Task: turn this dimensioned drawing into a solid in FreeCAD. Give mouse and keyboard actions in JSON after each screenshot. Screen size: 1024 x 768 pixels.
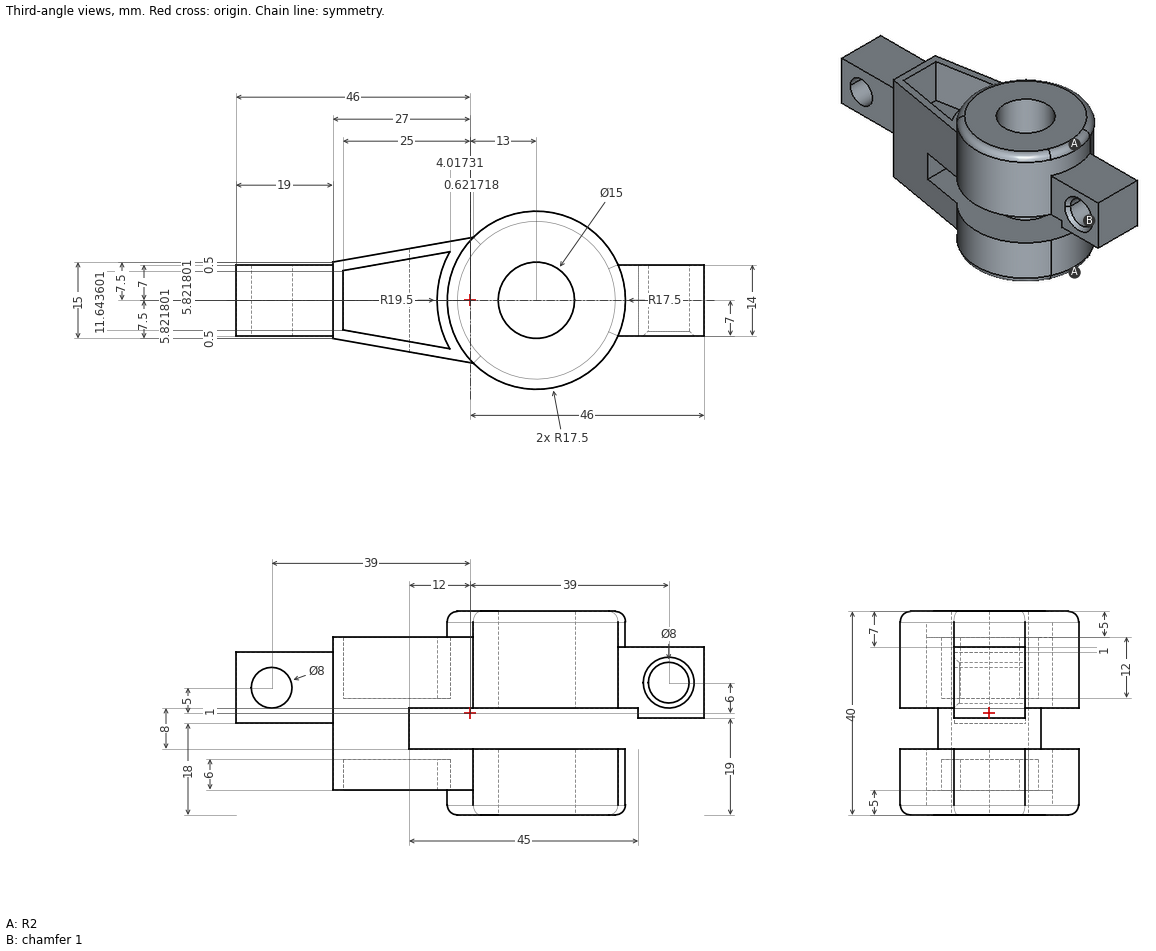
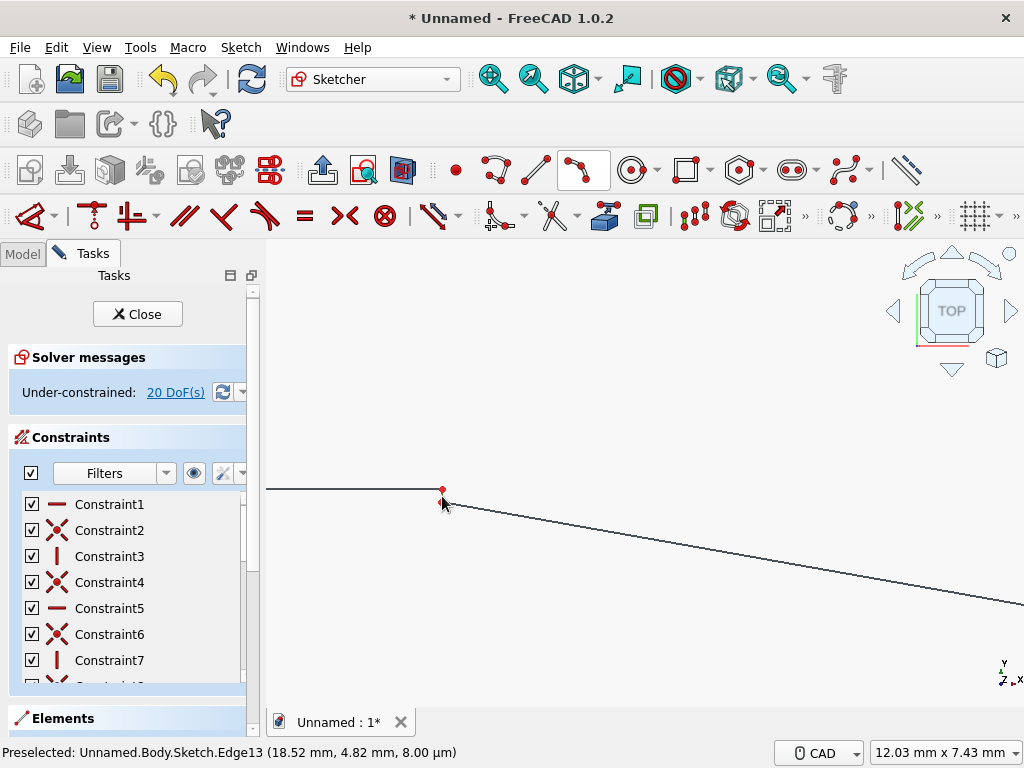
{"action": "left_click", "coordinate": [158, 216]}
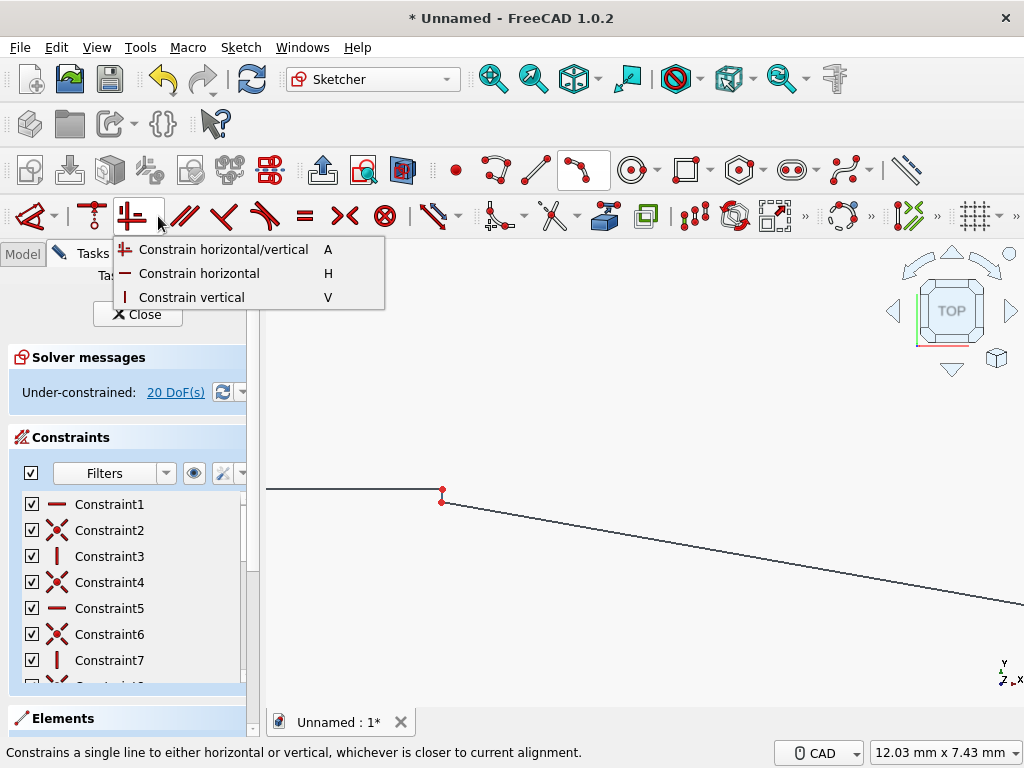
{"action": "left_click", "coordinate": [249, 297]}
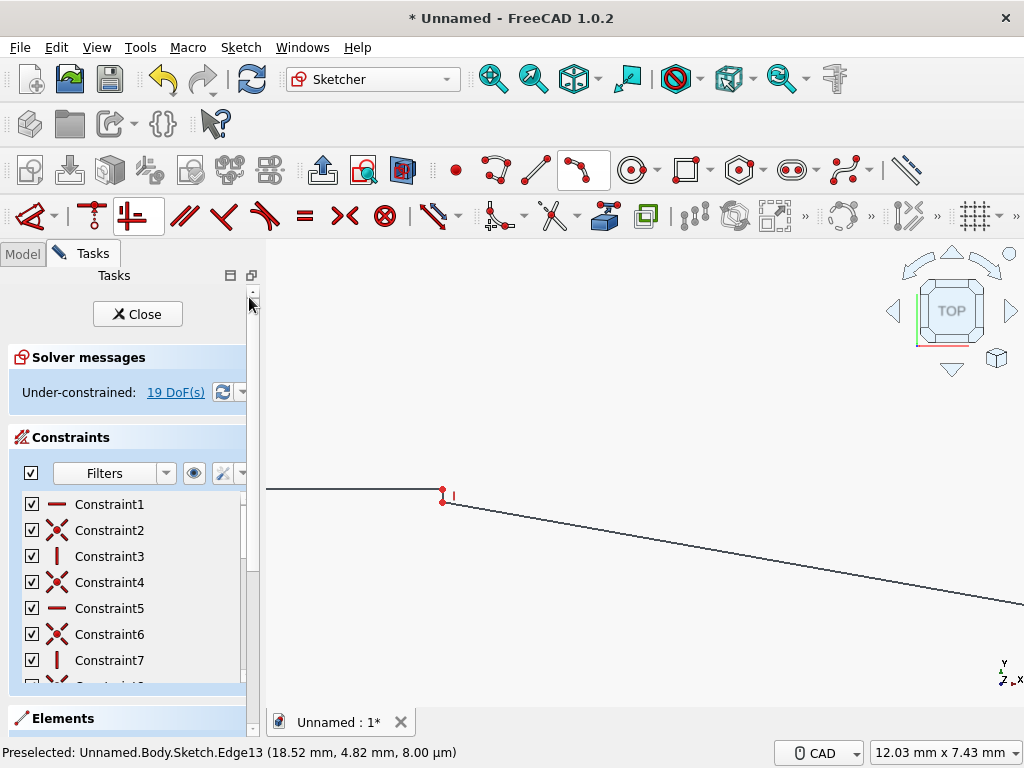
{"action": "scroll", "coordinate": [451, 509], "scroll_direction": "down", "scroll_amount": 13}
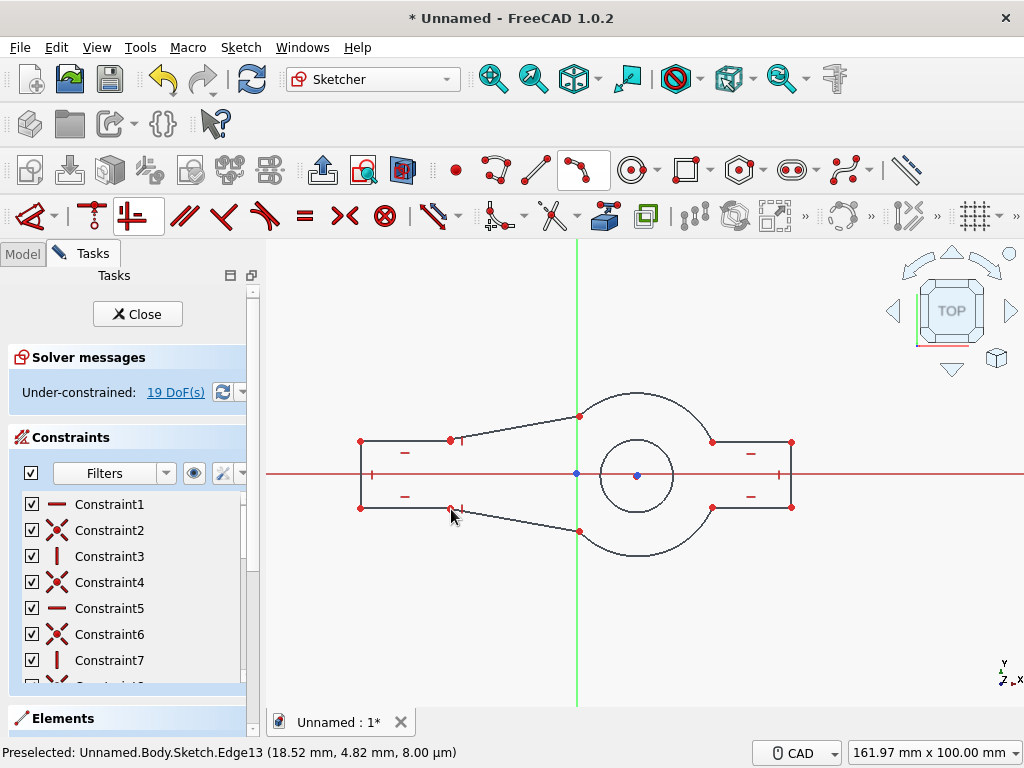
{"action": "left_click", "coordinate": [662, 450]}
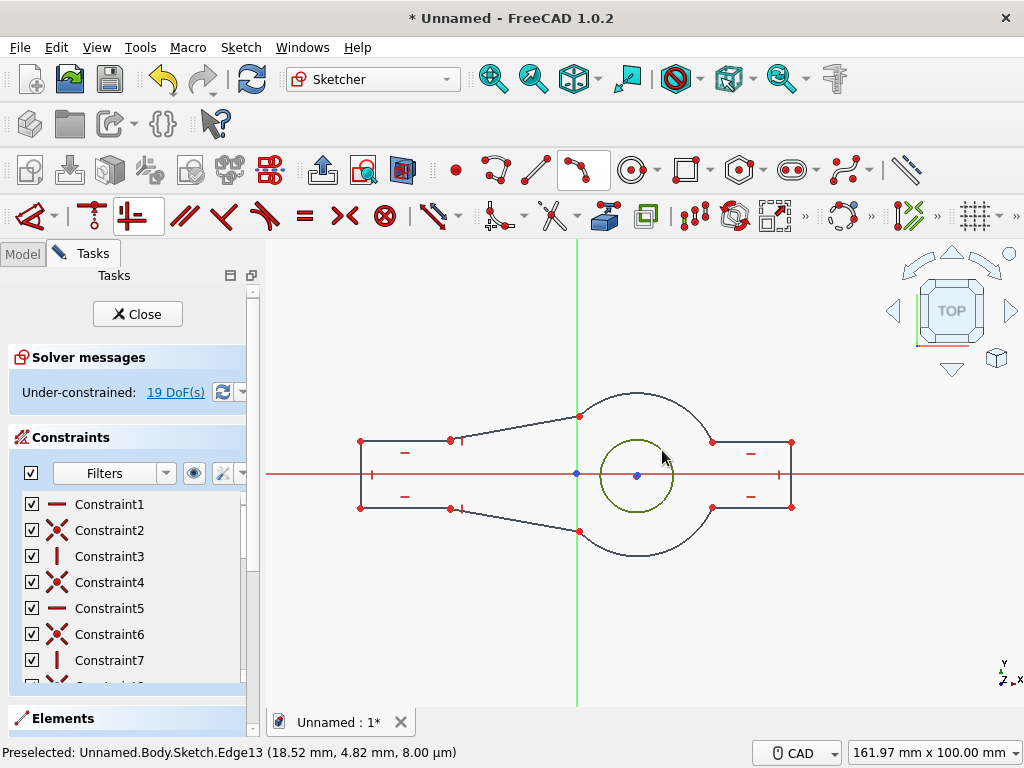
{"action": "left_click", "coordinate": [621, 555]}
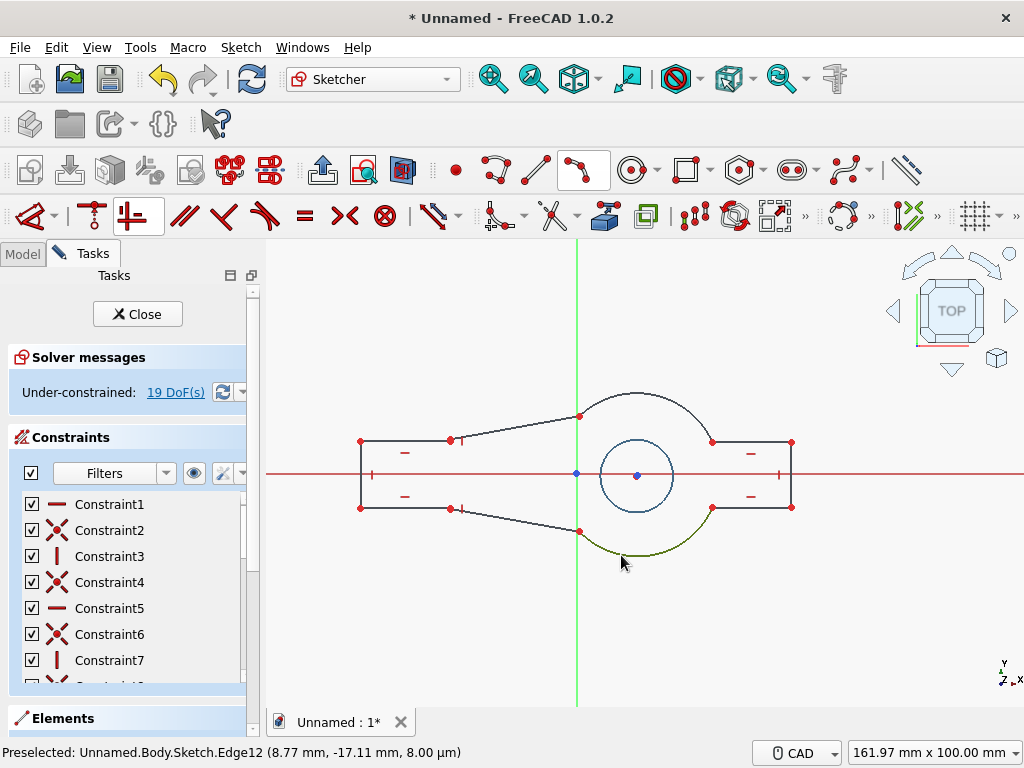
{"action": "left_click", "coordinate": [92, 216]}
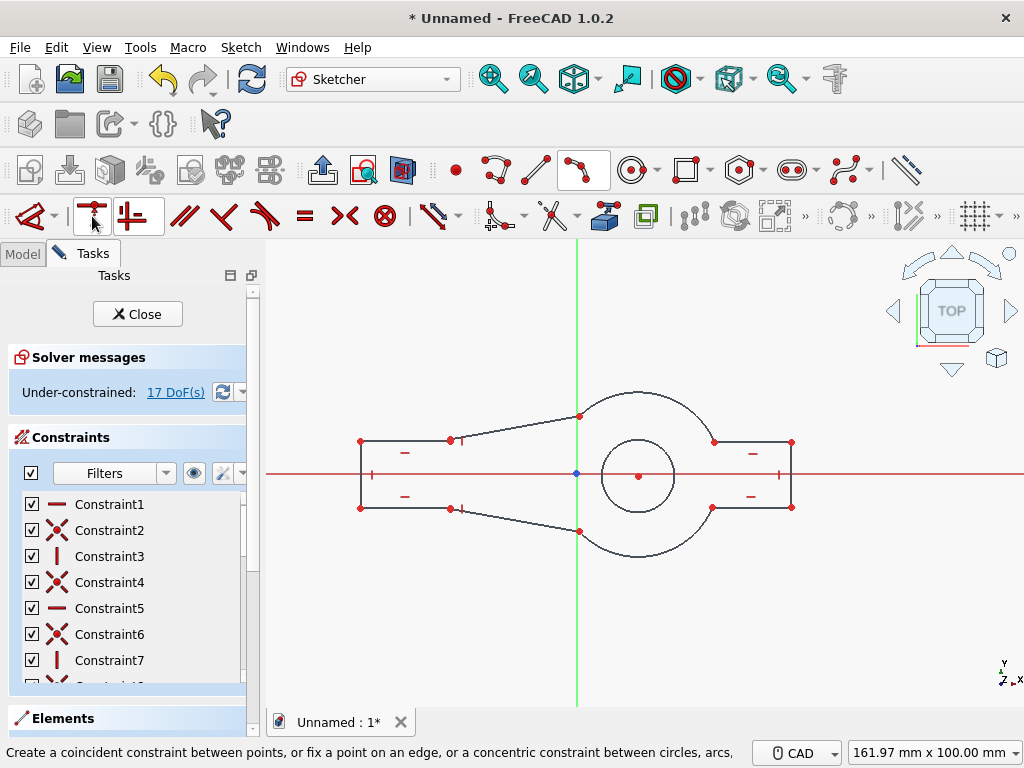
{"action": "left_click", "coordinate": [684, 406]}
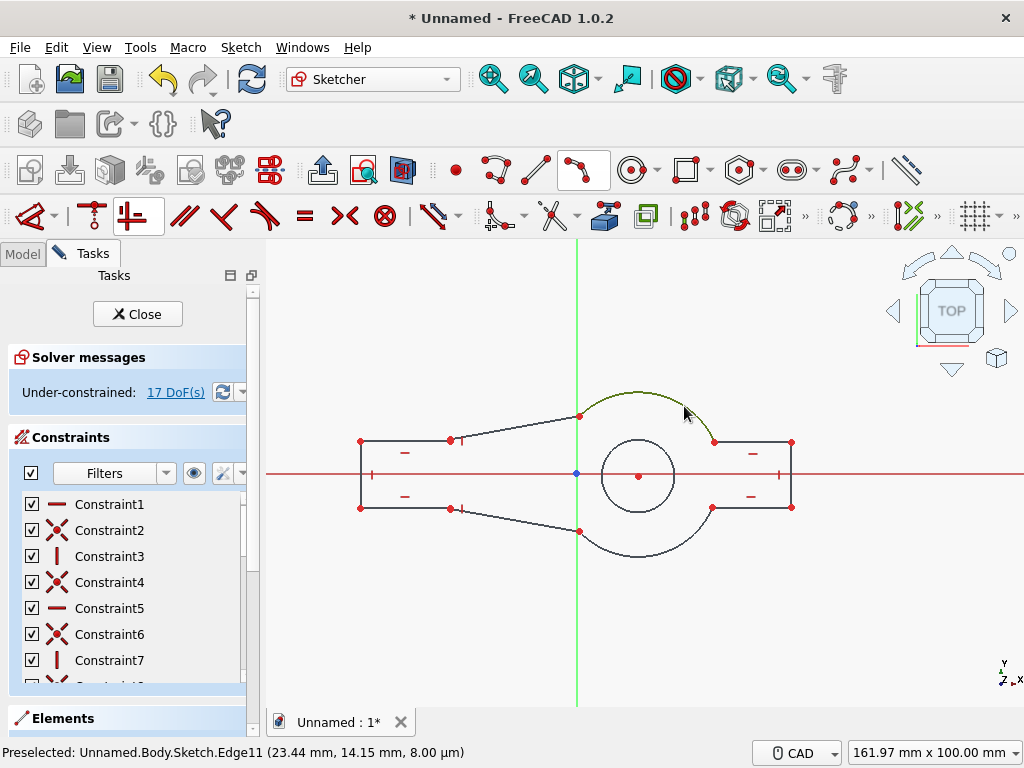
{"action": "left_click", "coordinate": [621, 555]}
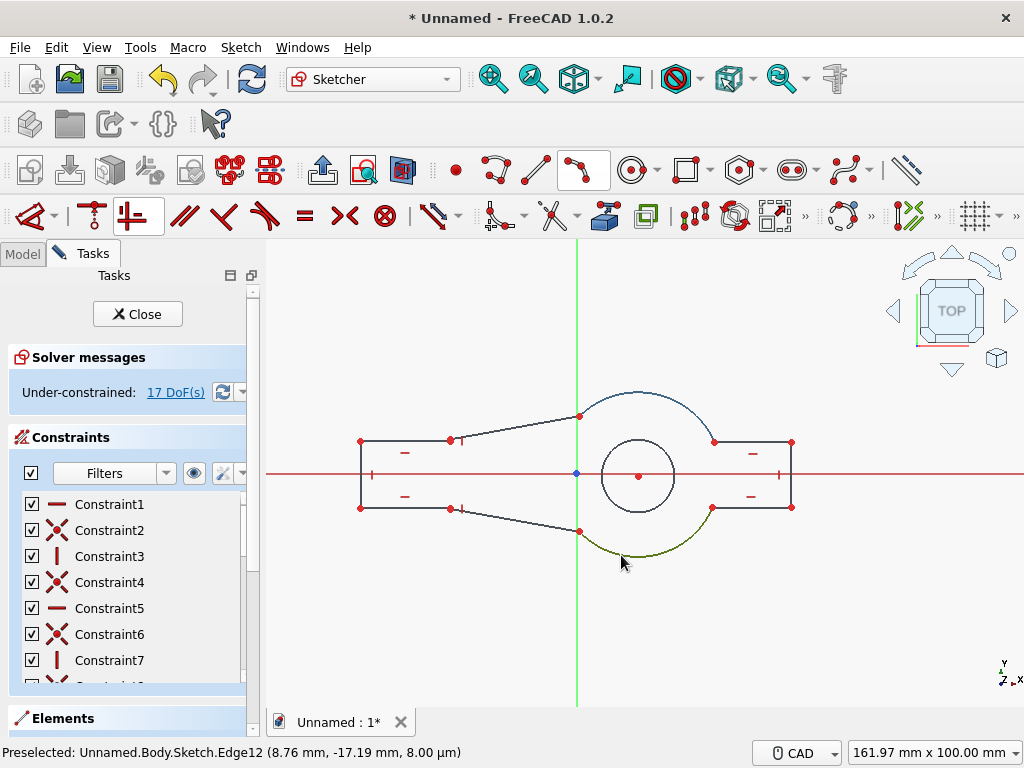
{"action": "left_click", "coordinate": [306, 216]}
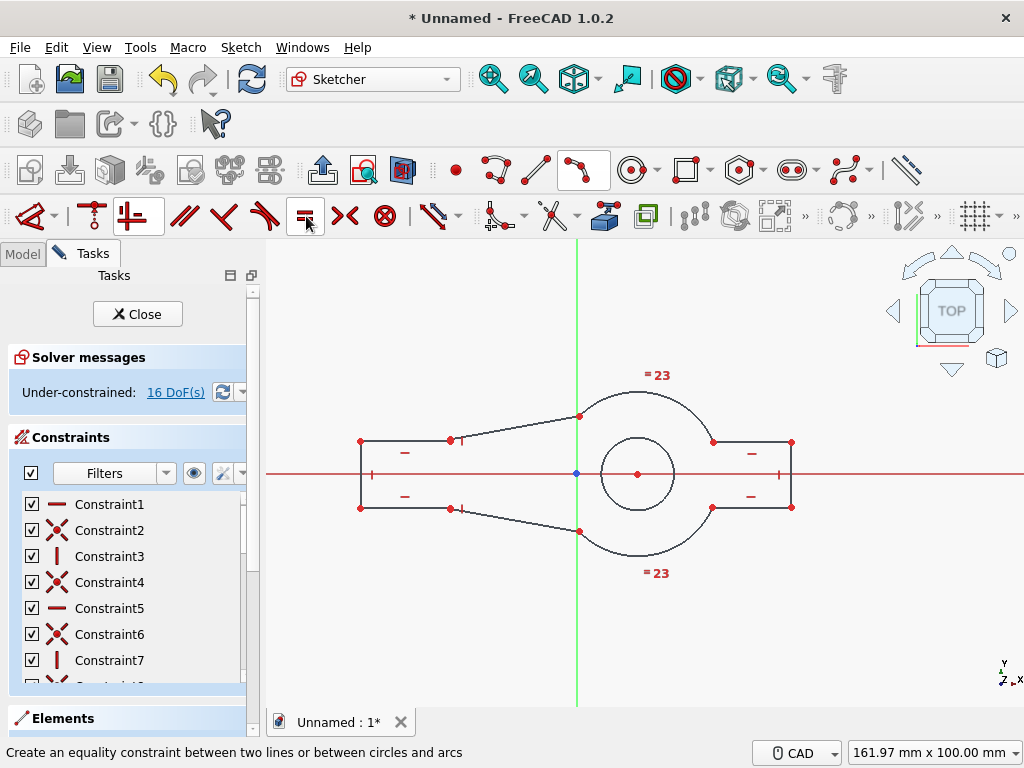
{"action": "left_click", "coordinate": [638, 474]}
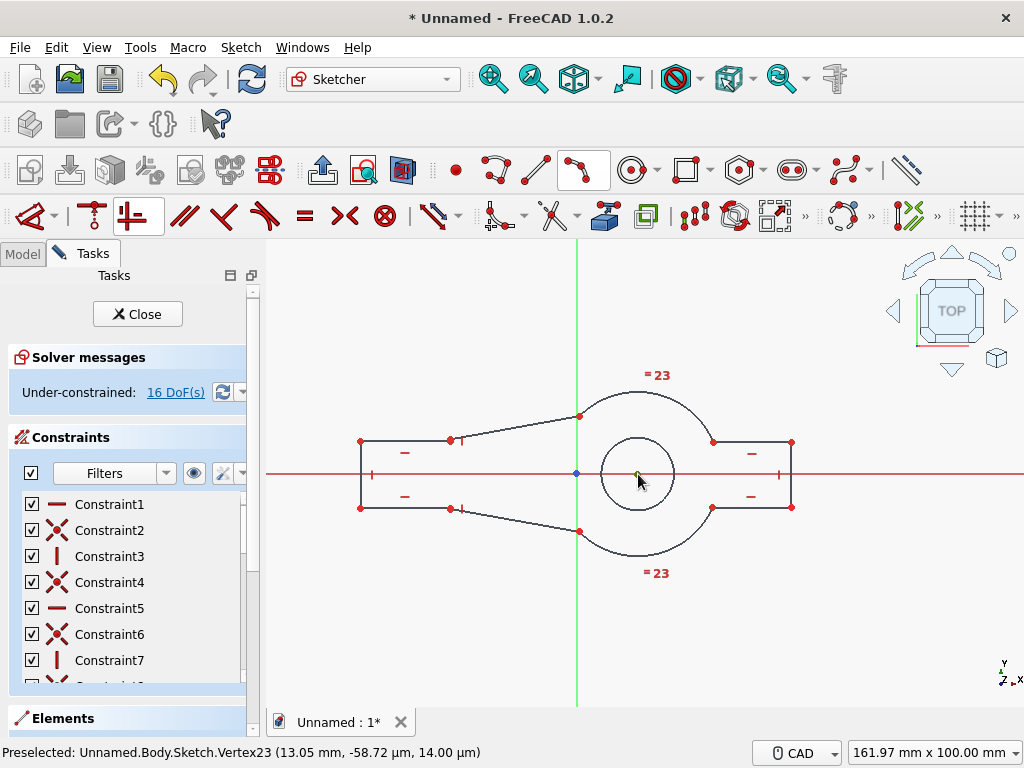
{"action": "left_click", "coordinate": [415, 474]}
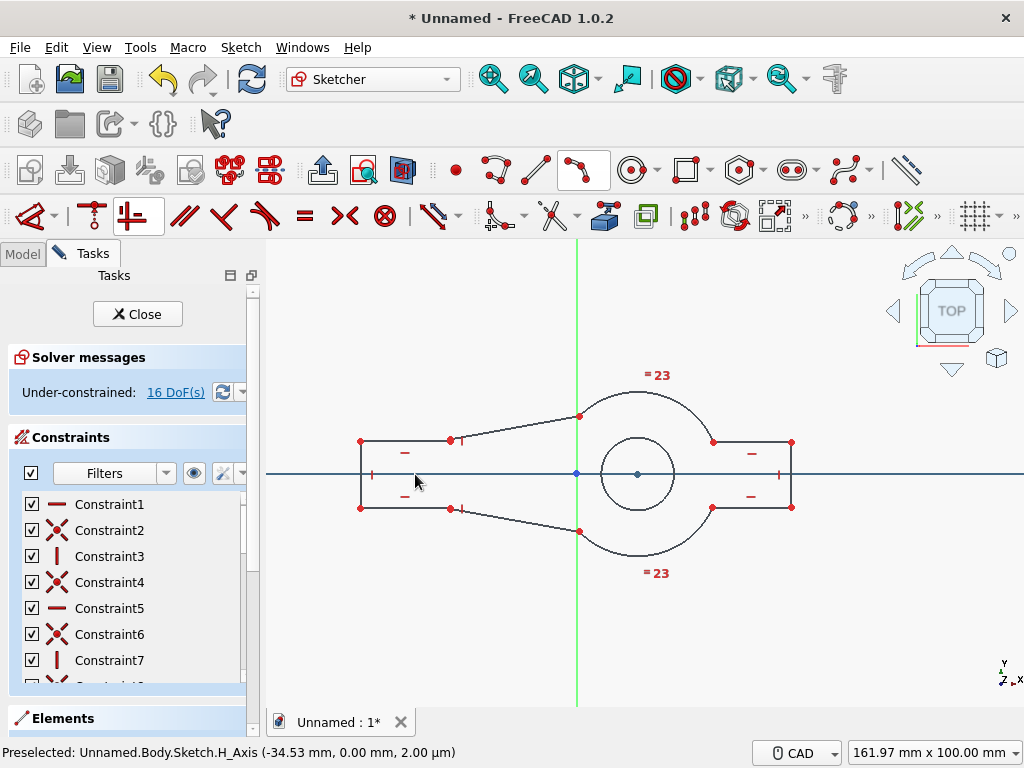
{"action": "left_click", "coordinate": [92, 216]}